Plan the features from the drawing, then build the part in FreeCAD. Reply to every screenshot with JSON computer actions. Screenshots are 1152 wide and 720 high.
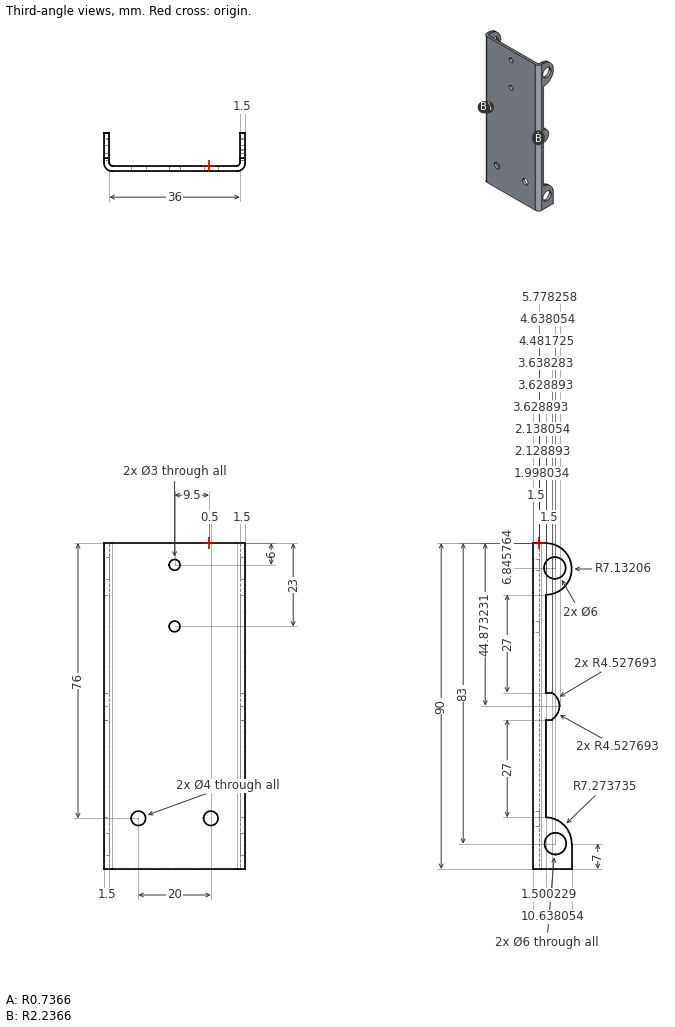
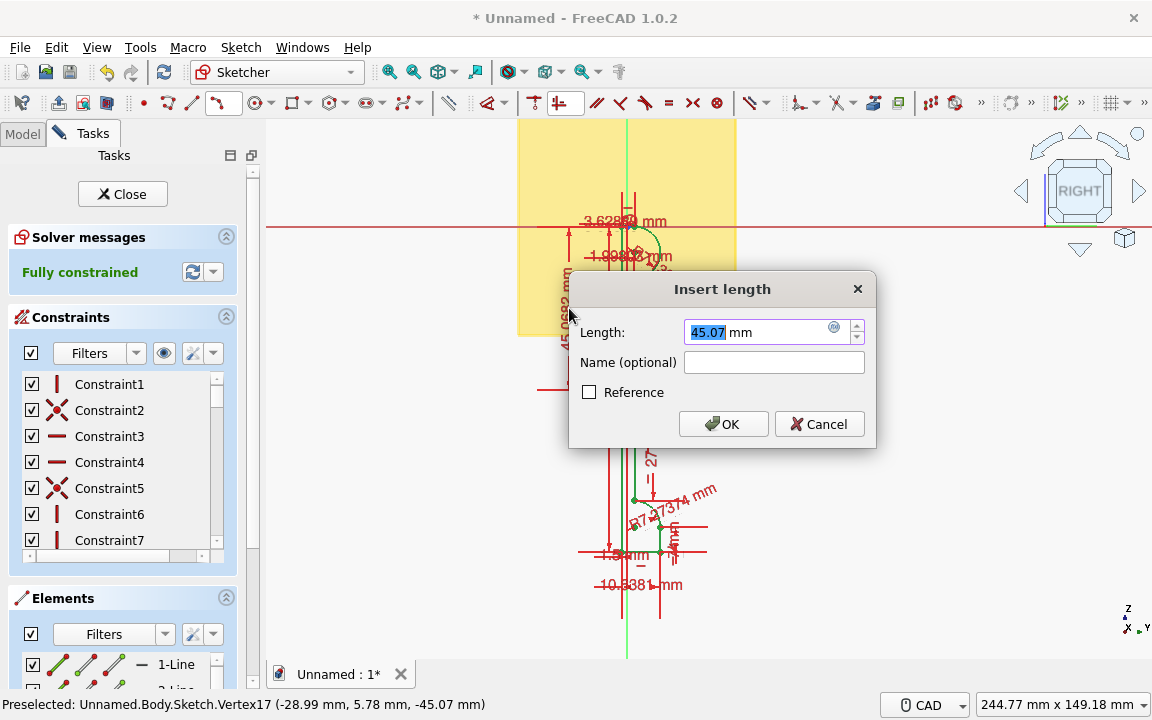
{"action": "type", "text": "44.873231"}
{"action": "key", "text": "Return"}
{"action": "key", "text": "Escape"}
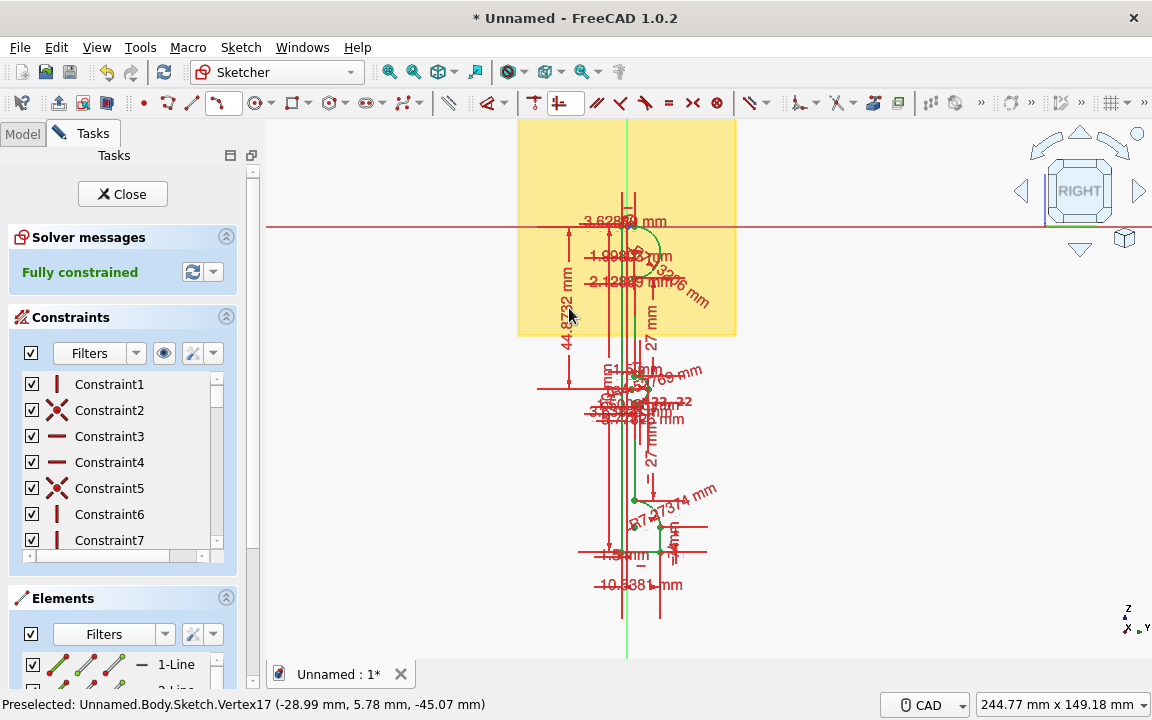
{"action": "left_click", "coordinate": [123, 194]}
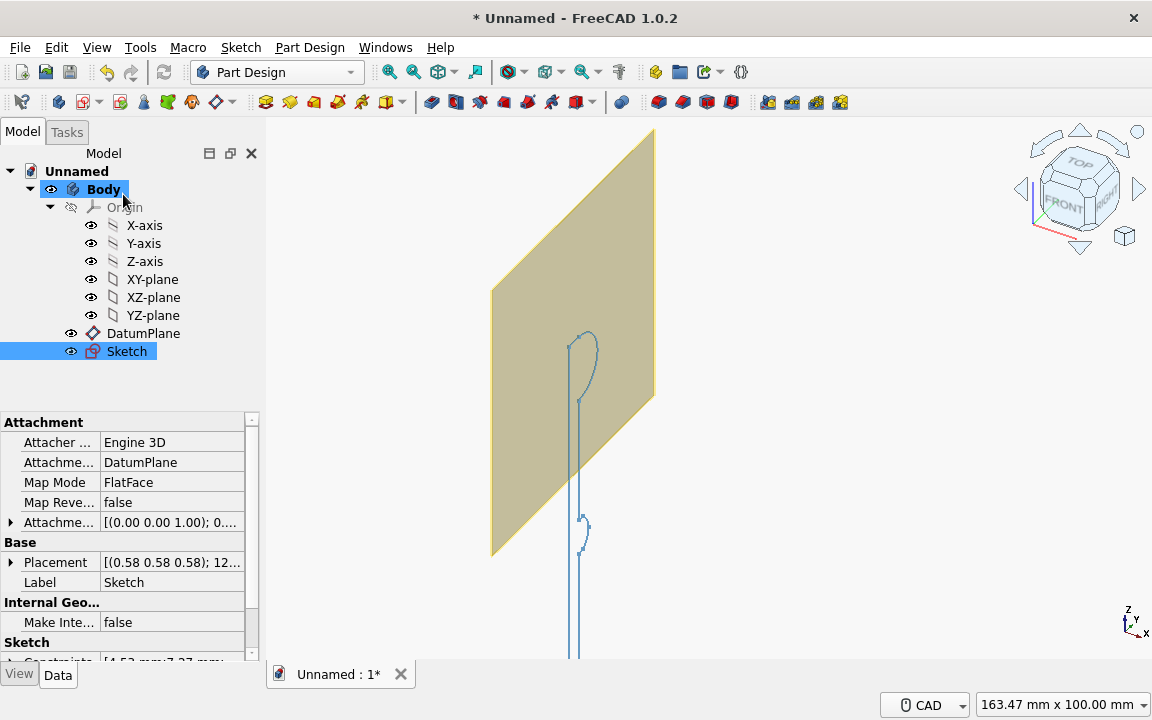
{"action": "left_click", "coordinate": [266, 102]}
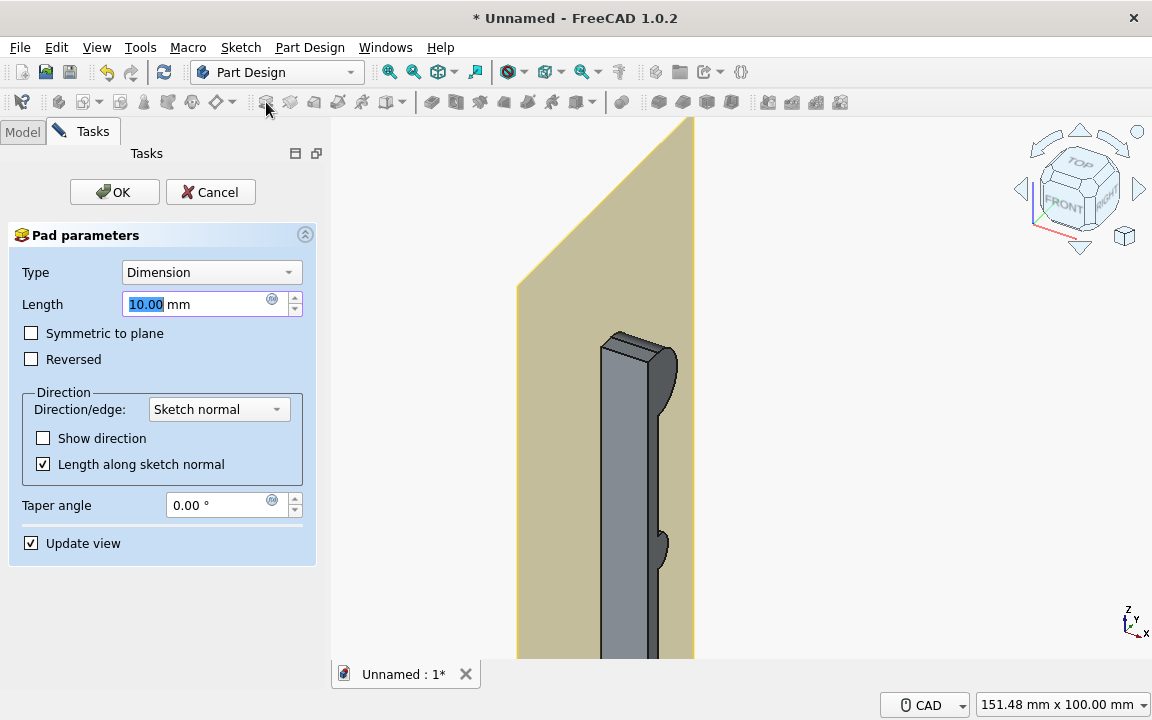
{"action": "type", "text": "1.5"}
{"action": "key", "text": "Tab"}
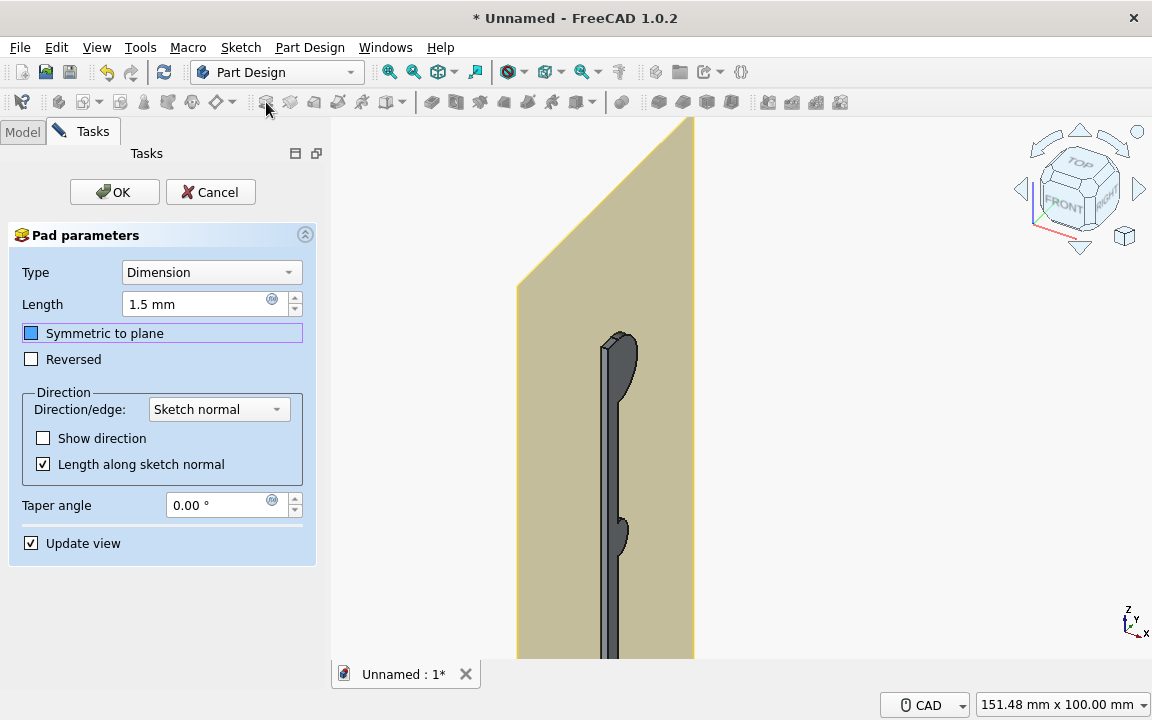
{"action": "left_click", "coordinate": [115, 192]}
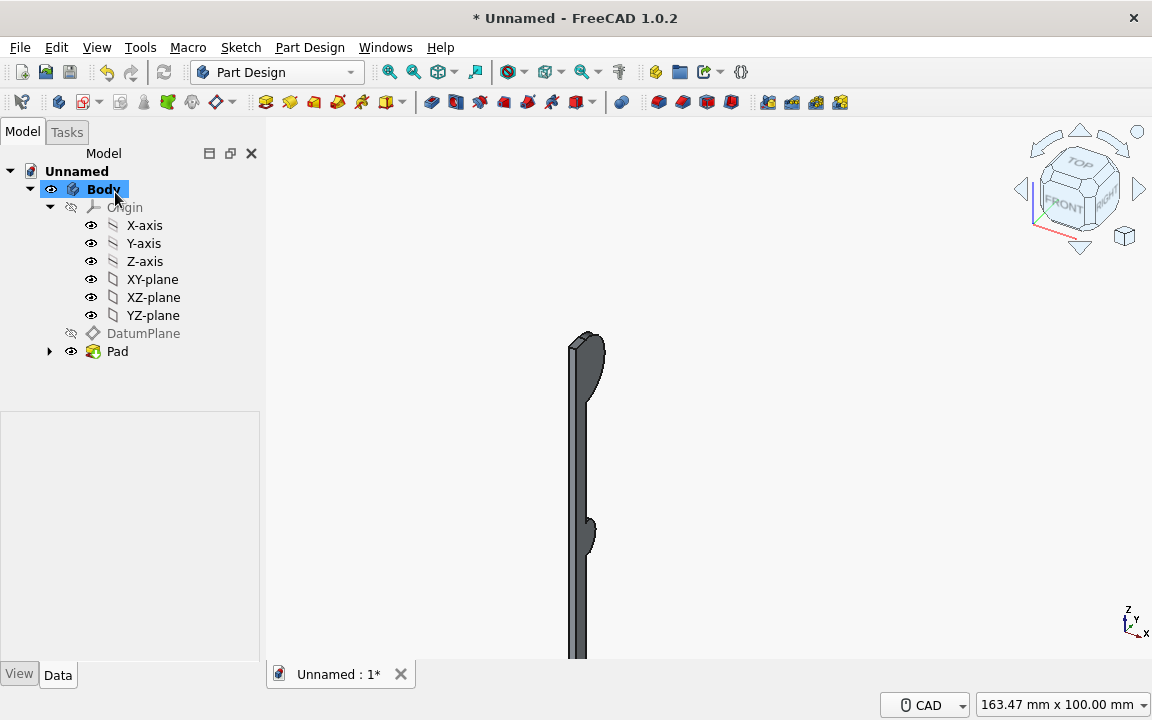
{"action": "key", "text": "v f"}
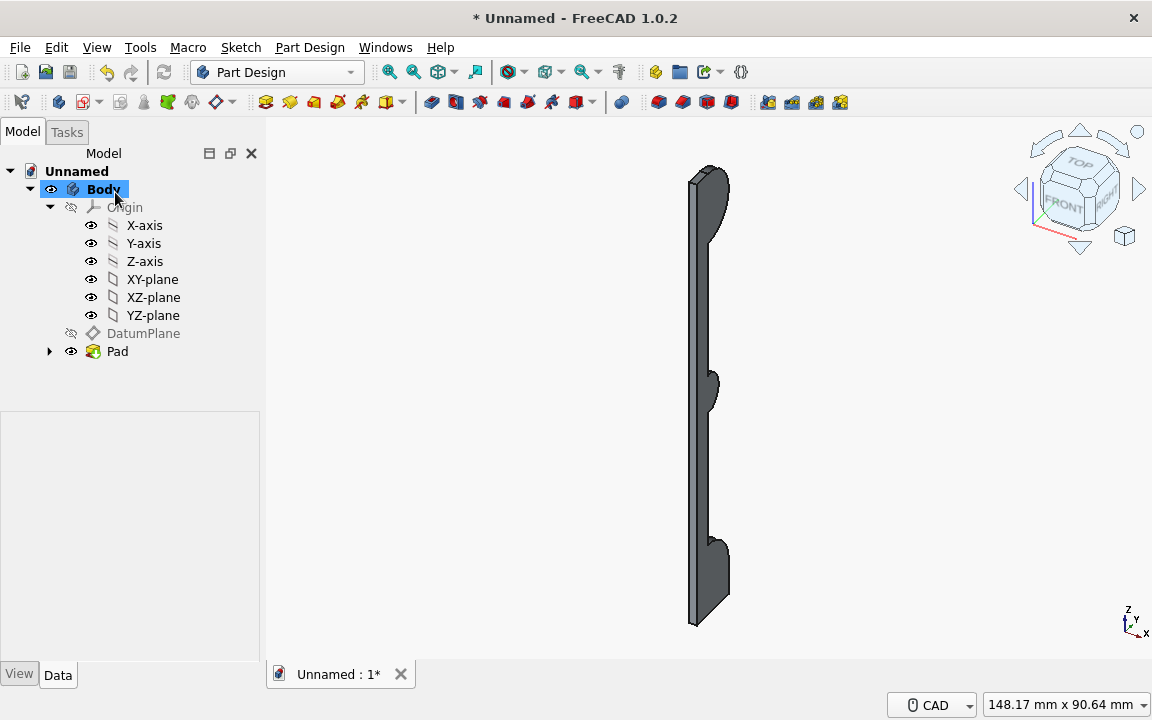
{"action": "left_click", "coordinate": [713, 577]}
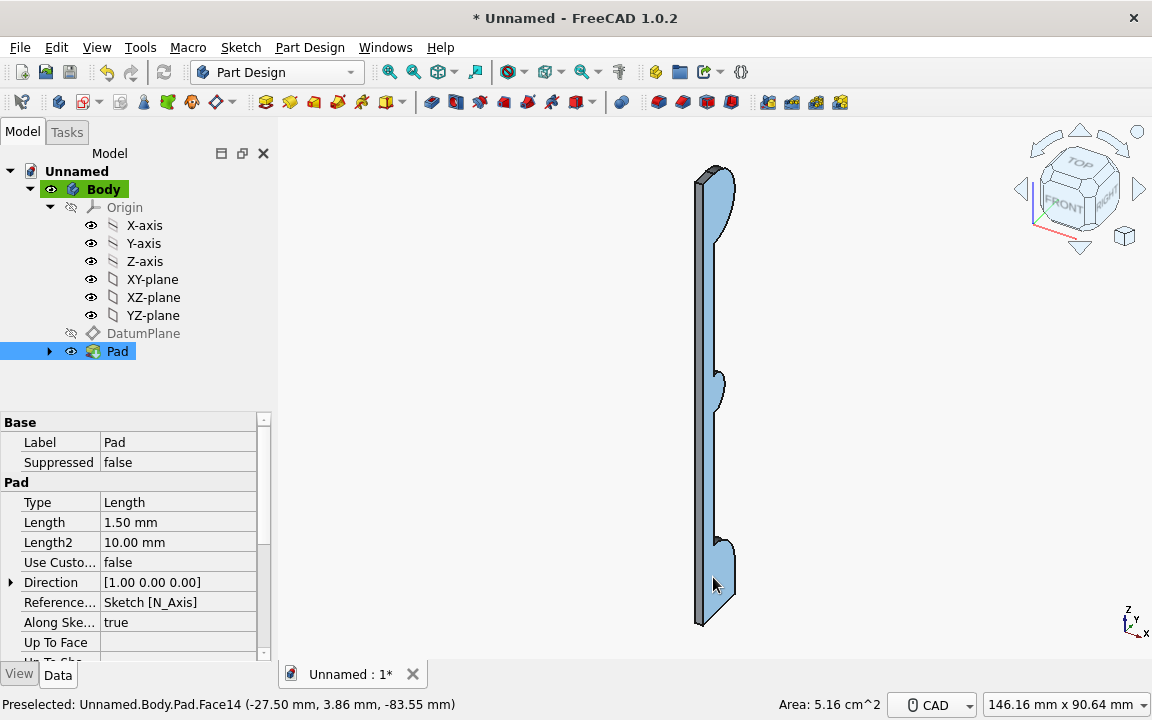
{"action": "left_click", "coordinate": [84, 102]}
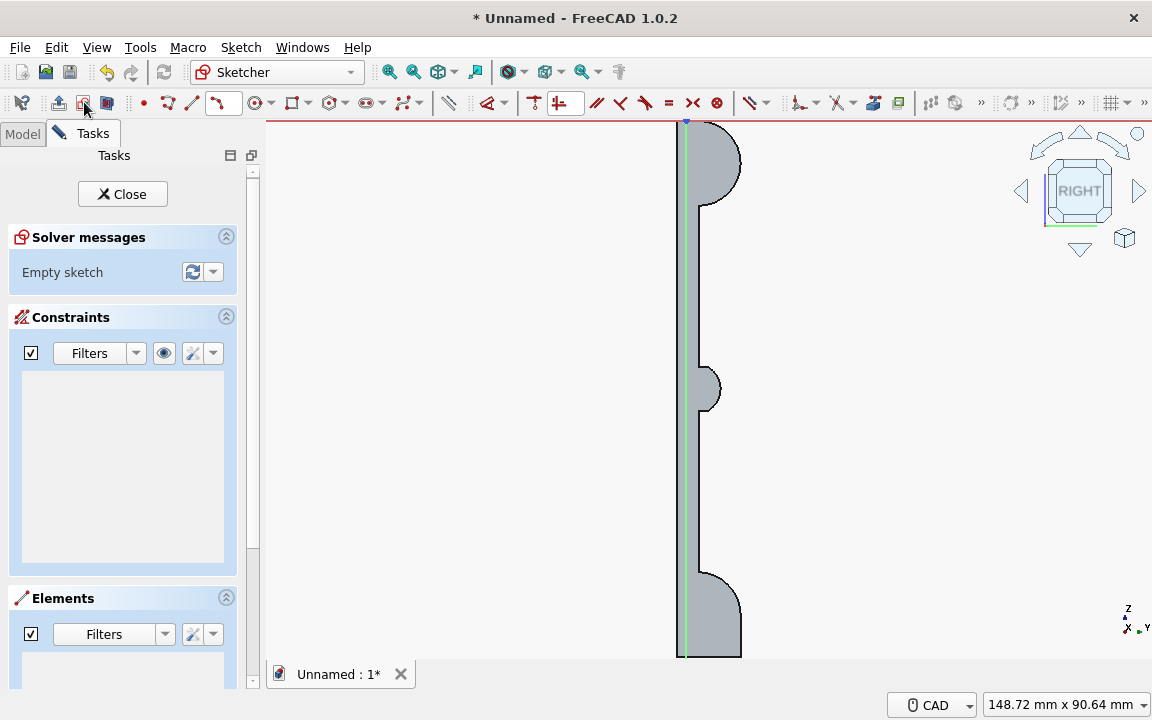
{"action": "scroll", "coordinate": [557, 389], "scroll_direction": "down", "scroll_amount": 2}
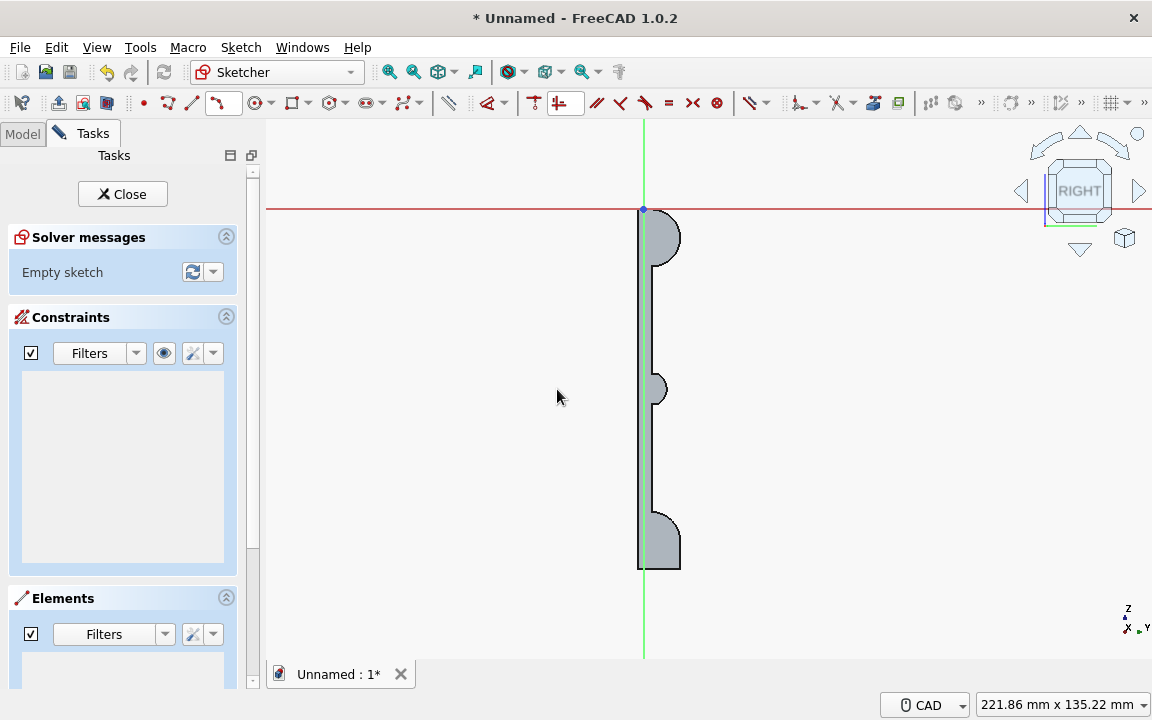
{"action": "left_click", "coordinate": [292, 104]}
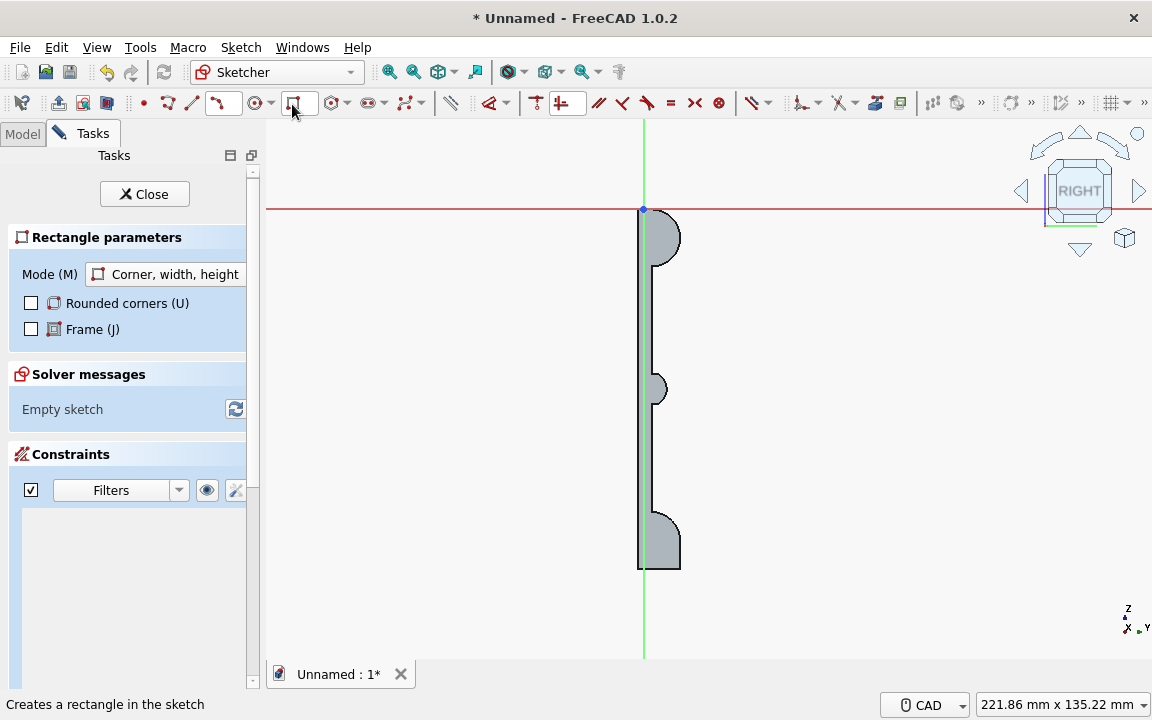
{"action": "scroll", "coordinate": [644, 209], "scroll_direction": "up", "scroll_amount": 5}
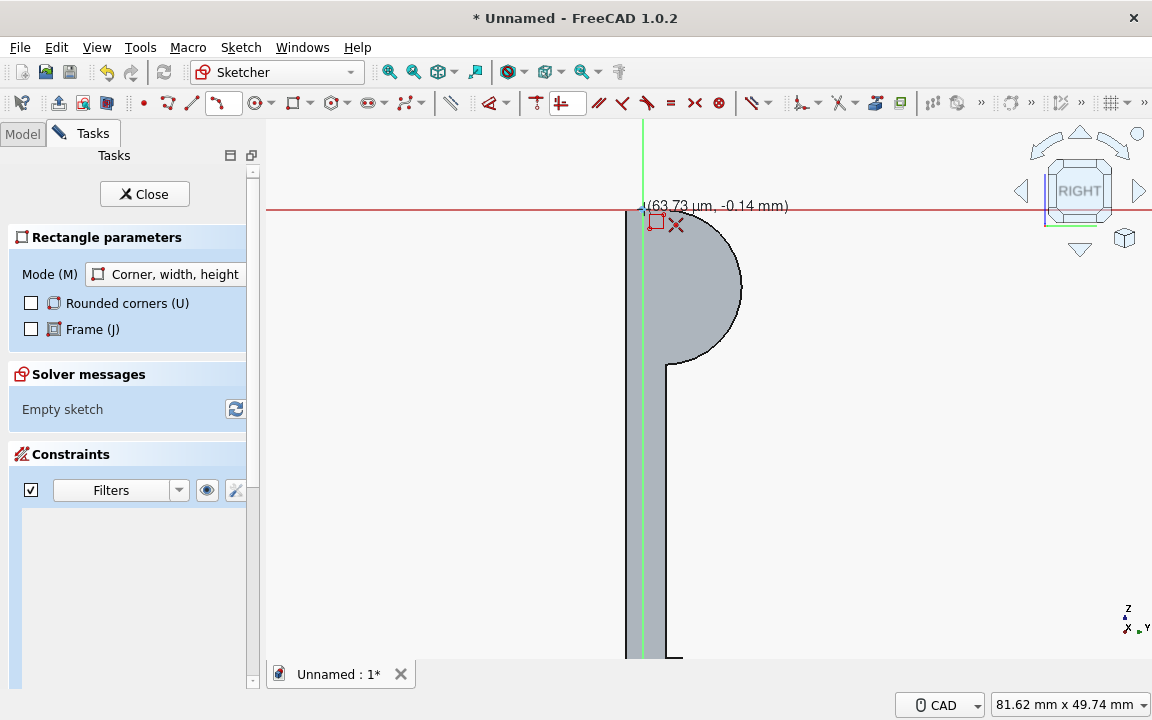
{"action": "left_click", "coordinate": [643, 210]}